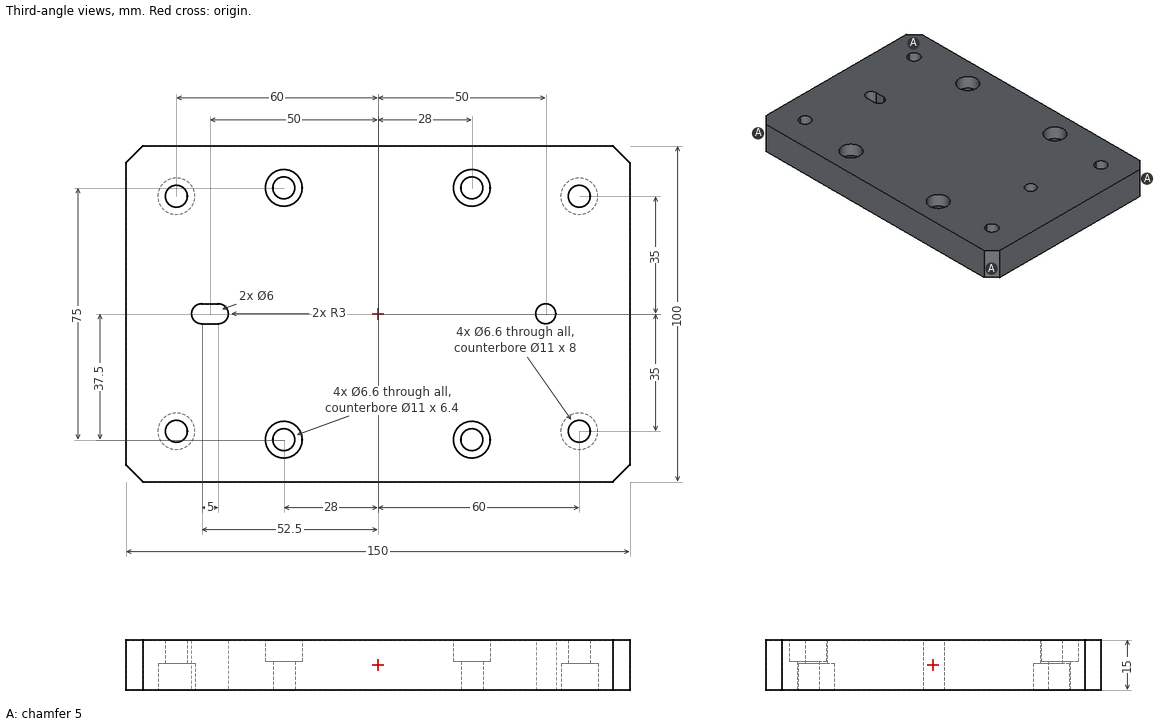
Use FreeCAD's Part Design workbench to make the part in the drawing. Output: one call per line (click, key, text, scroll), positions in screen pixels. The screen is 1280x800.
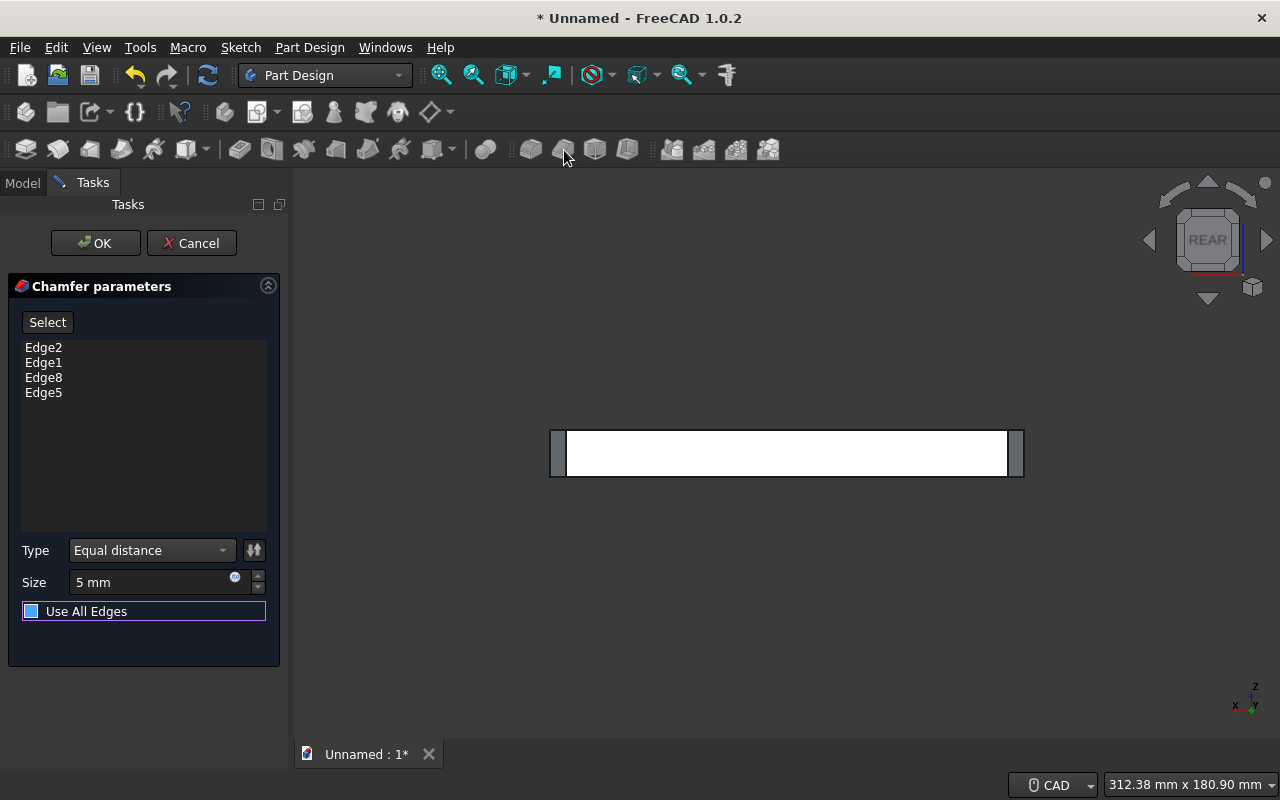
click(96, 243)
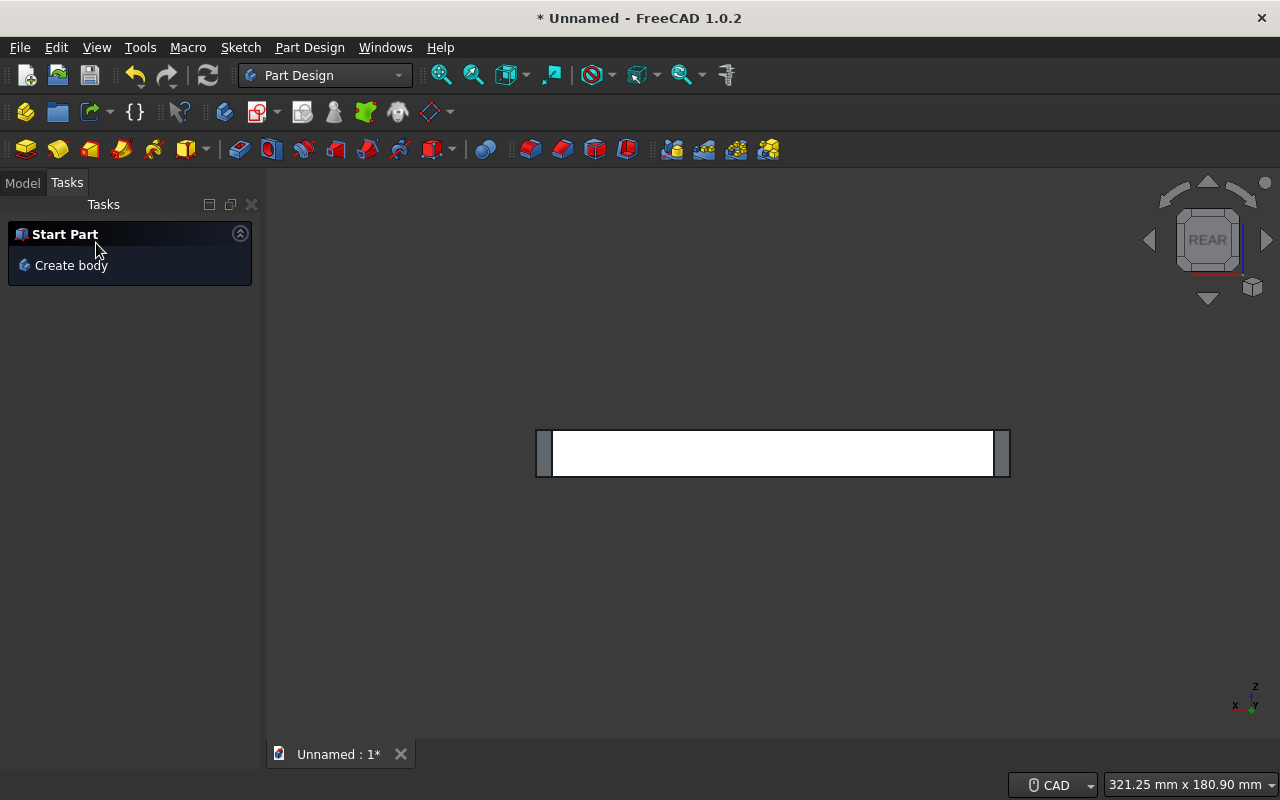
key(5)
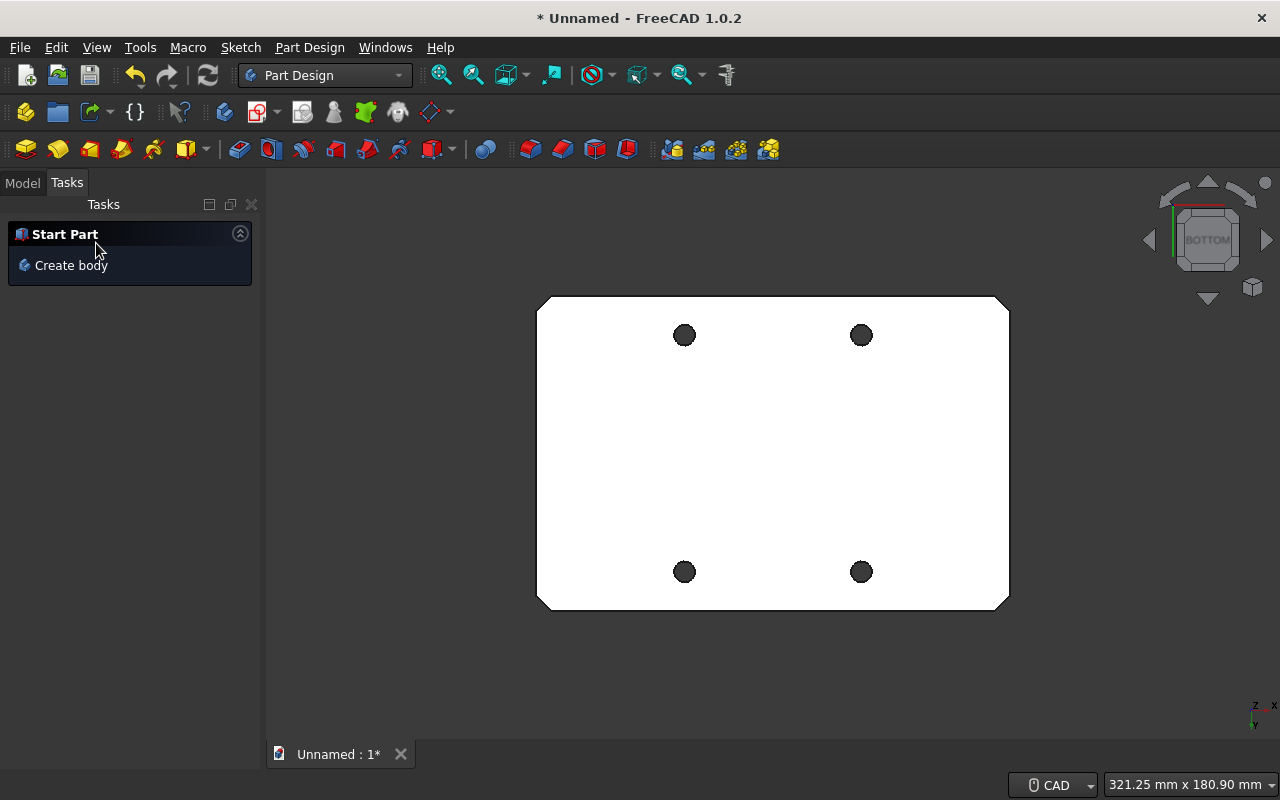
click(773, 452)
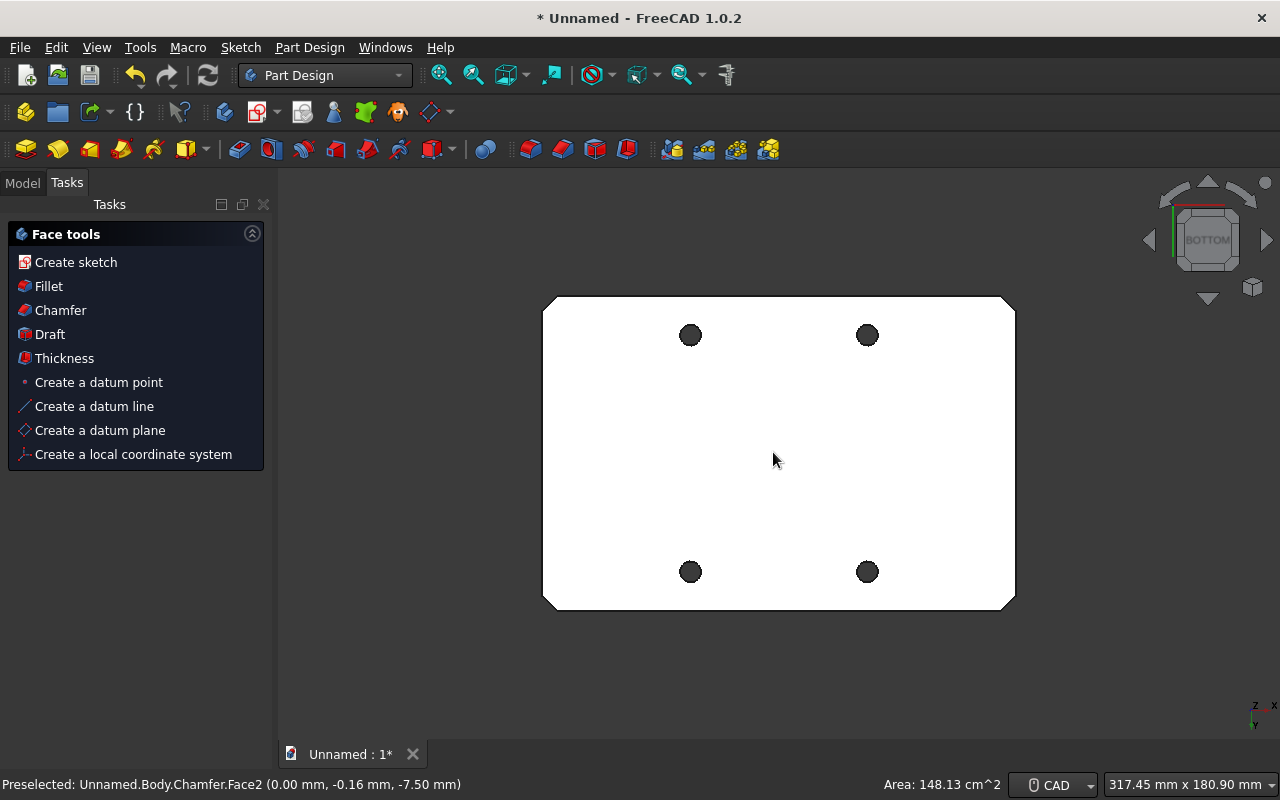
click(258, 112)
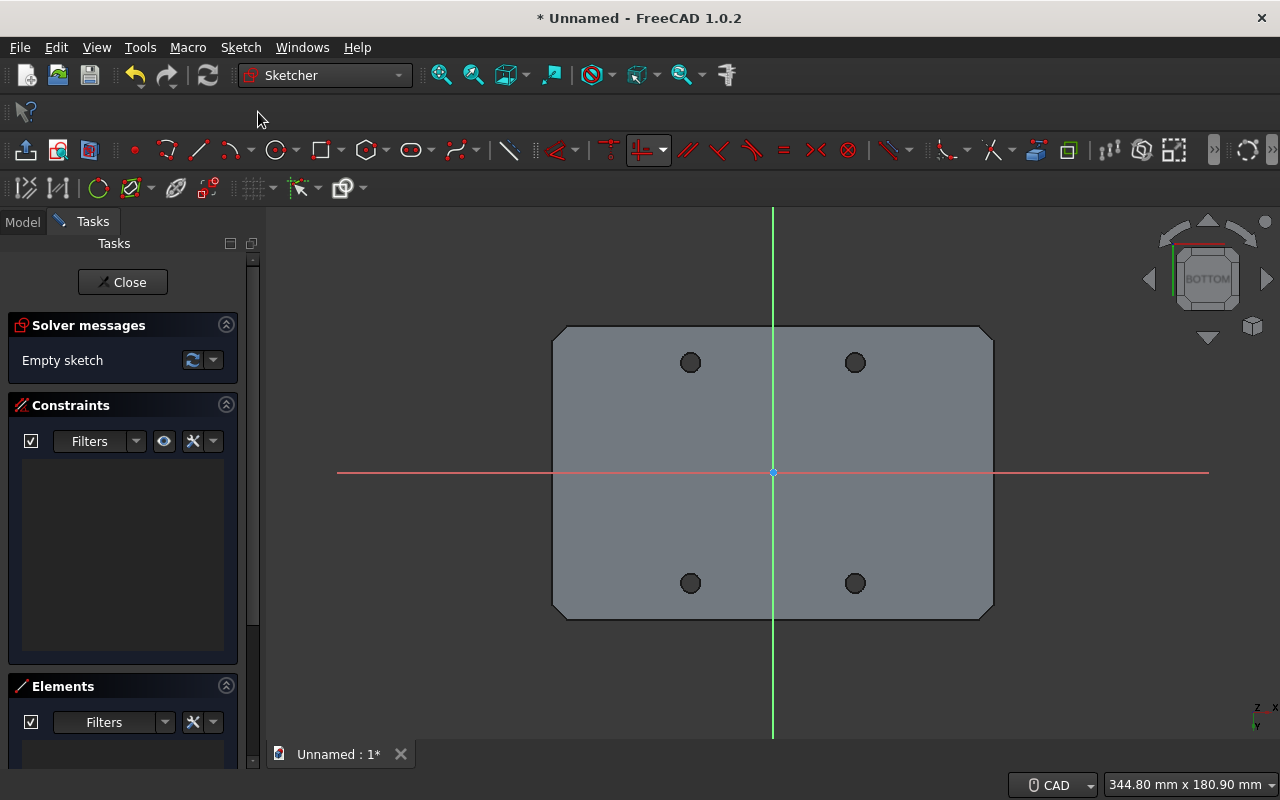
scroll(912, 473, up, 2)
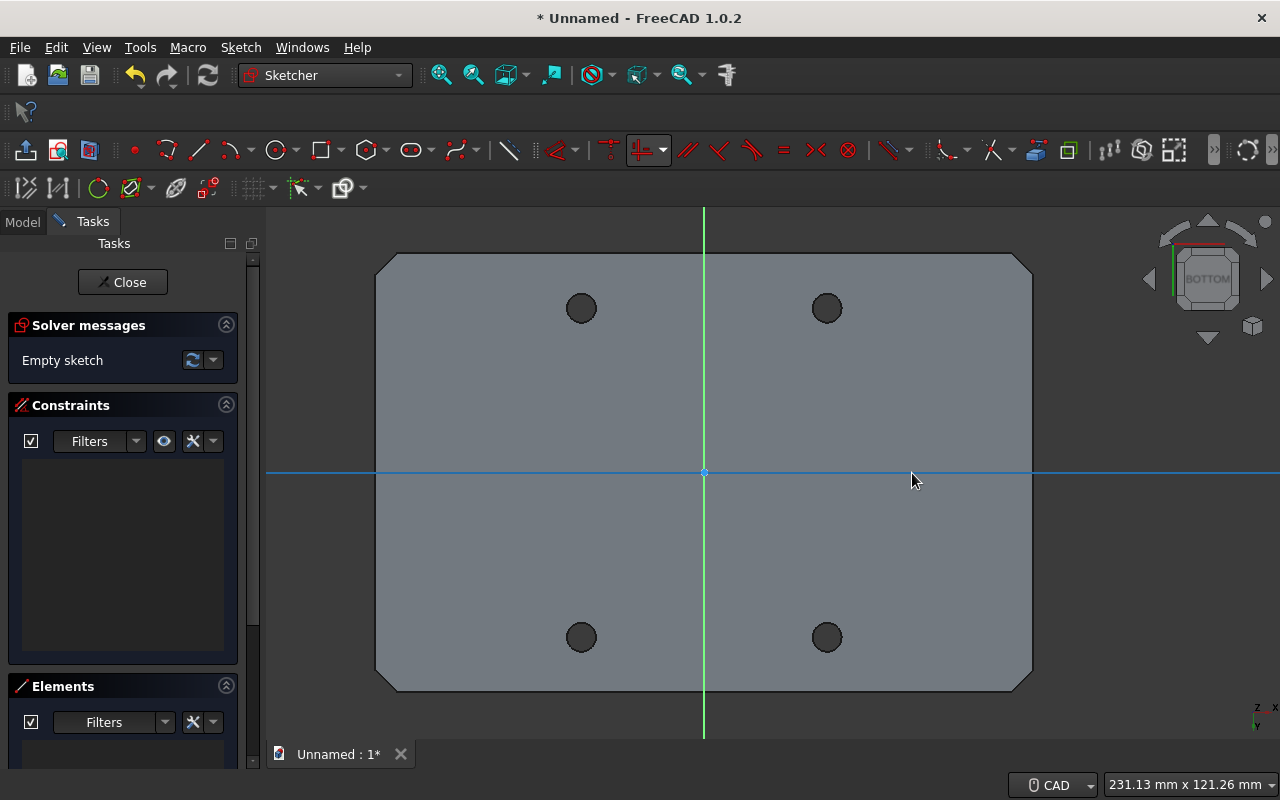
key(g)
key(c)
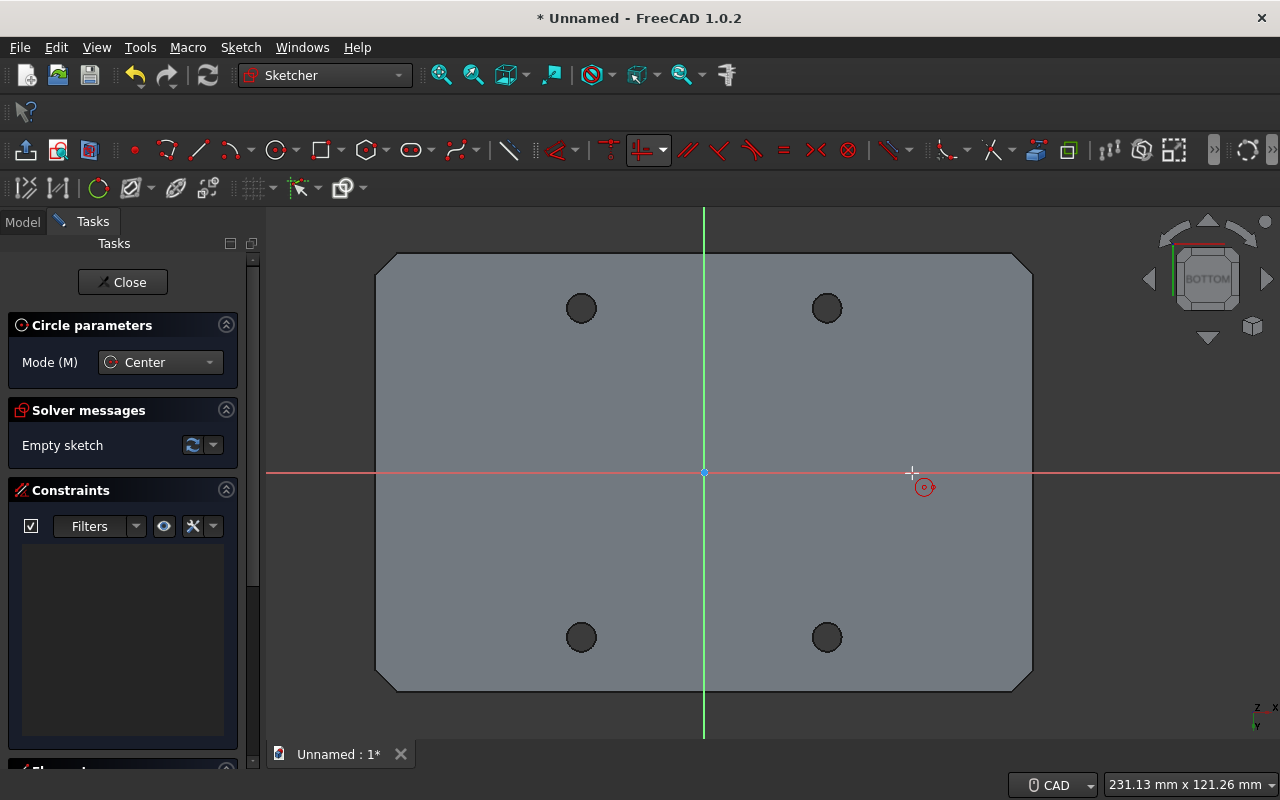
scroll(968, 319, up, 3)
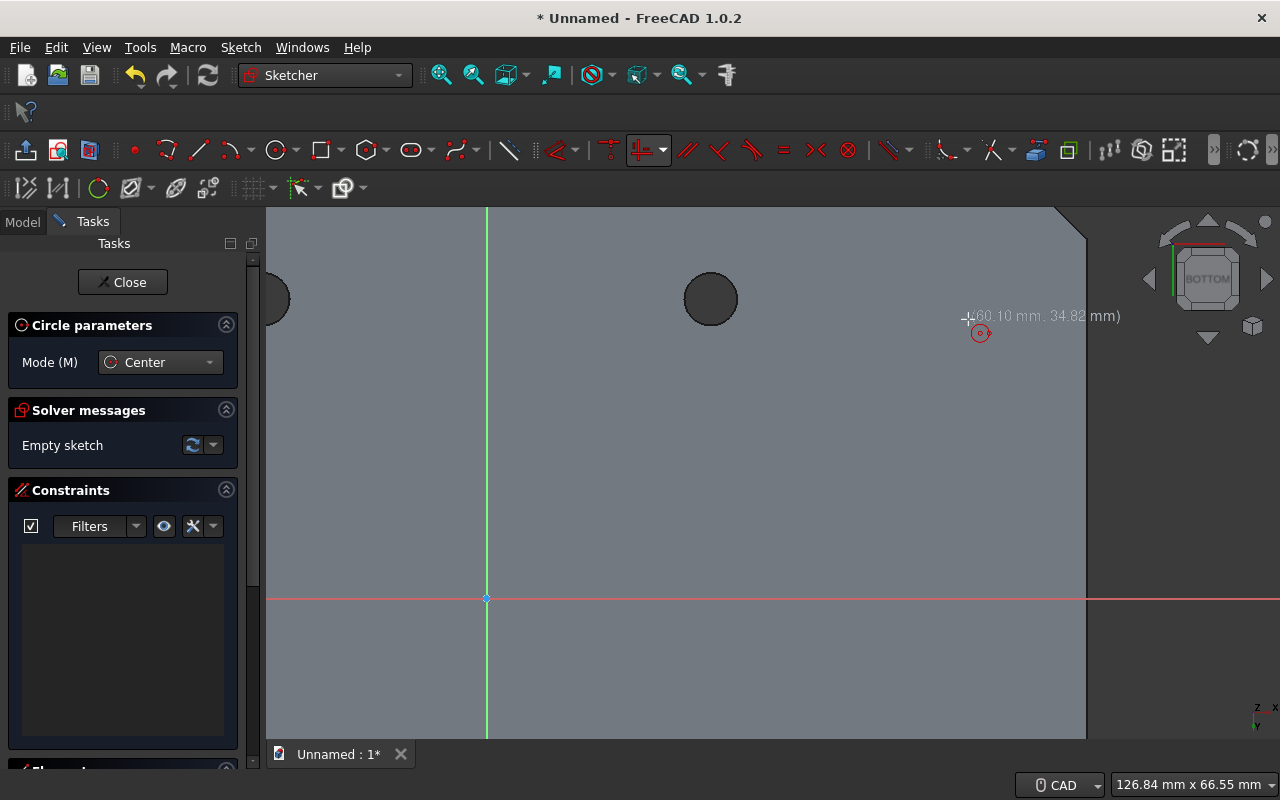
click(967, 319)
move(985, 301)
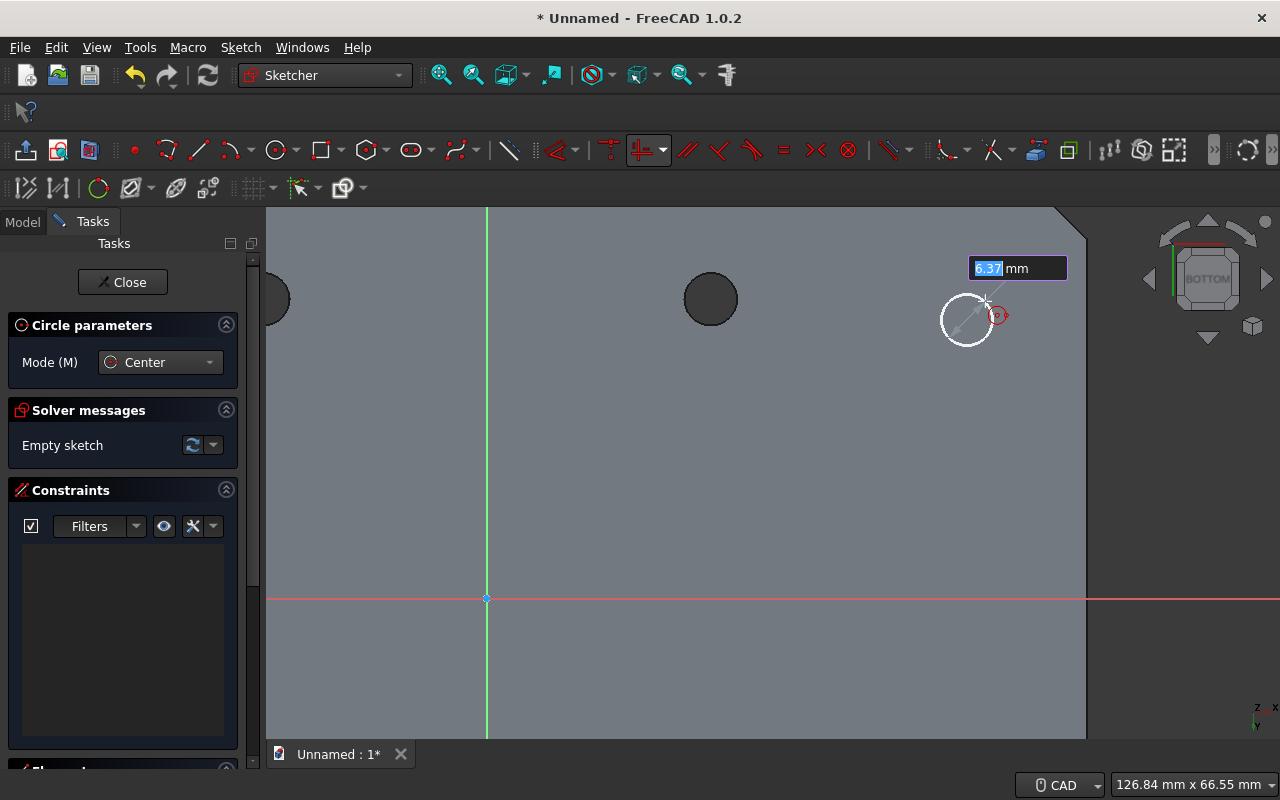
text(6.6)
key(Return)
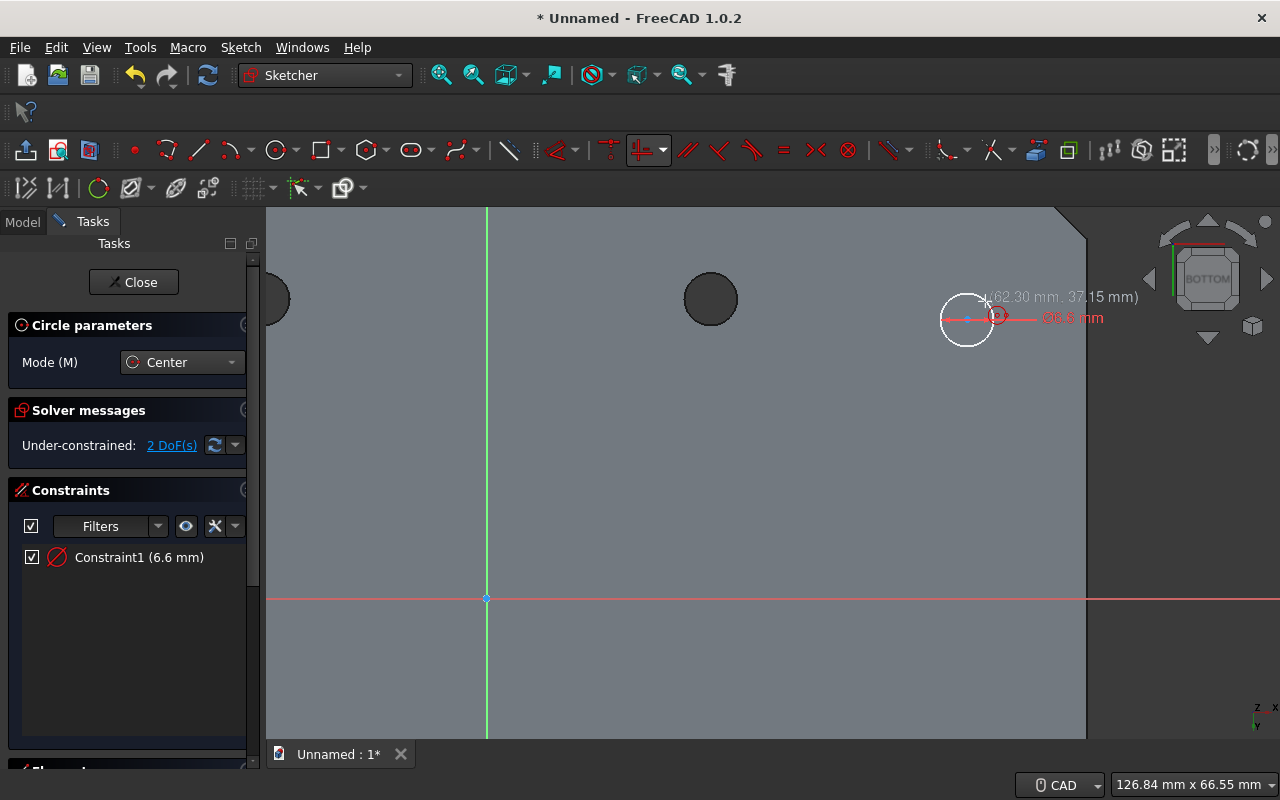
scroll(969, 320, down, 3)